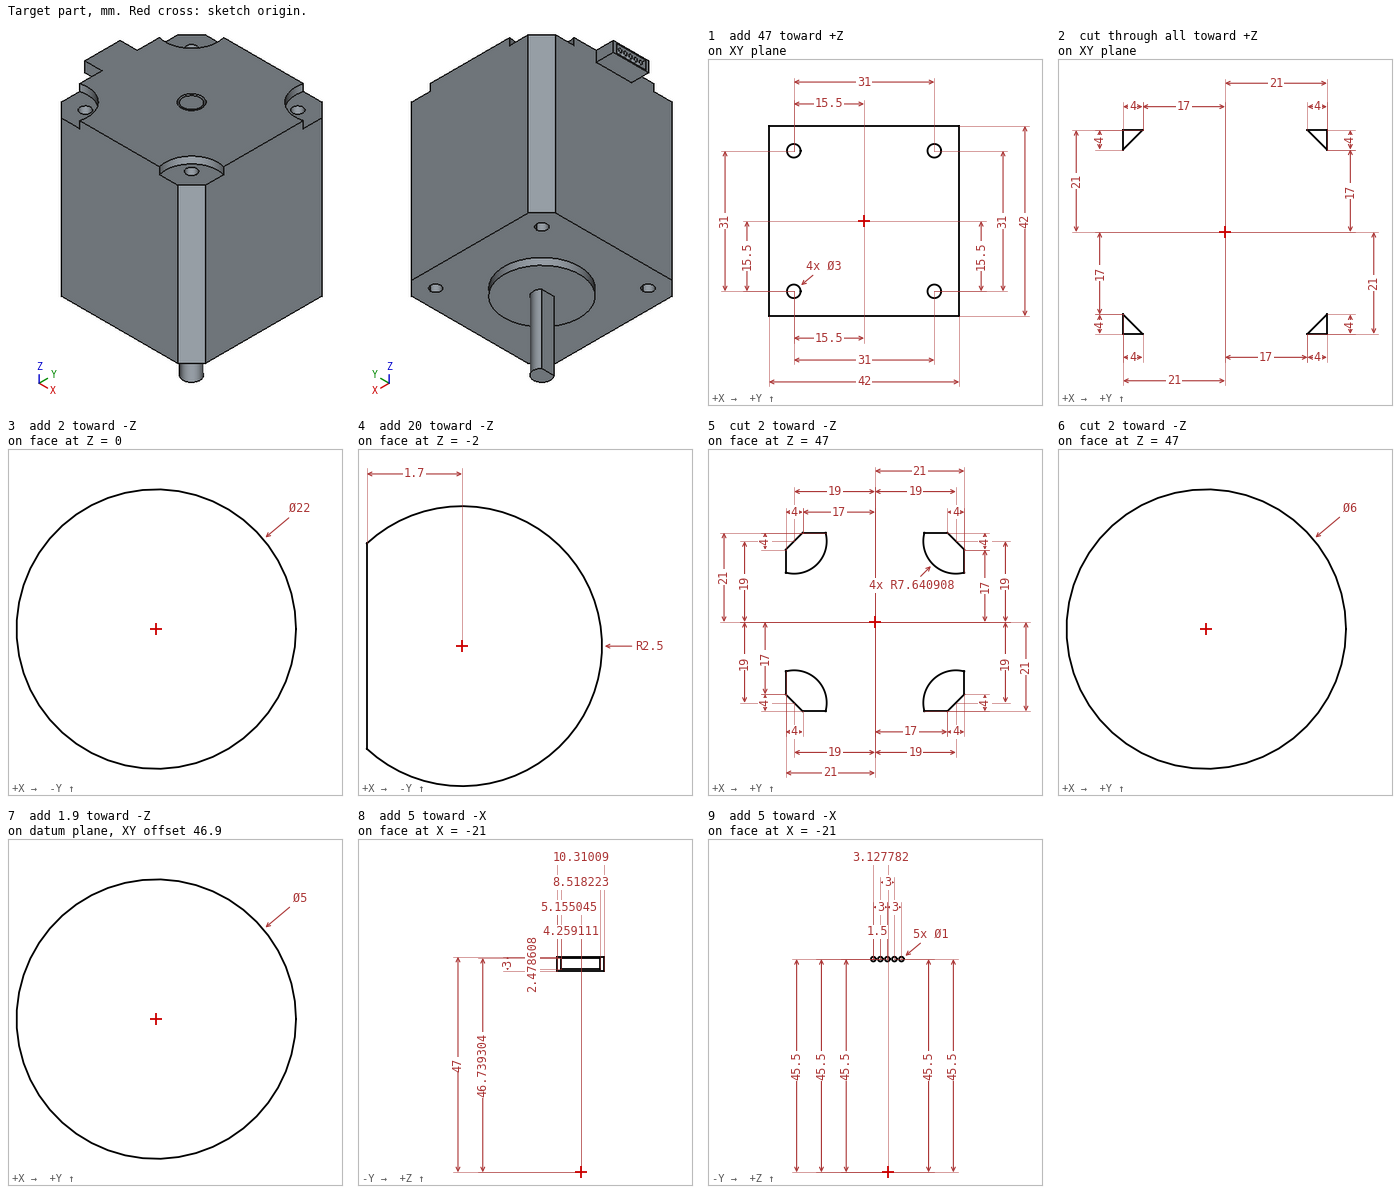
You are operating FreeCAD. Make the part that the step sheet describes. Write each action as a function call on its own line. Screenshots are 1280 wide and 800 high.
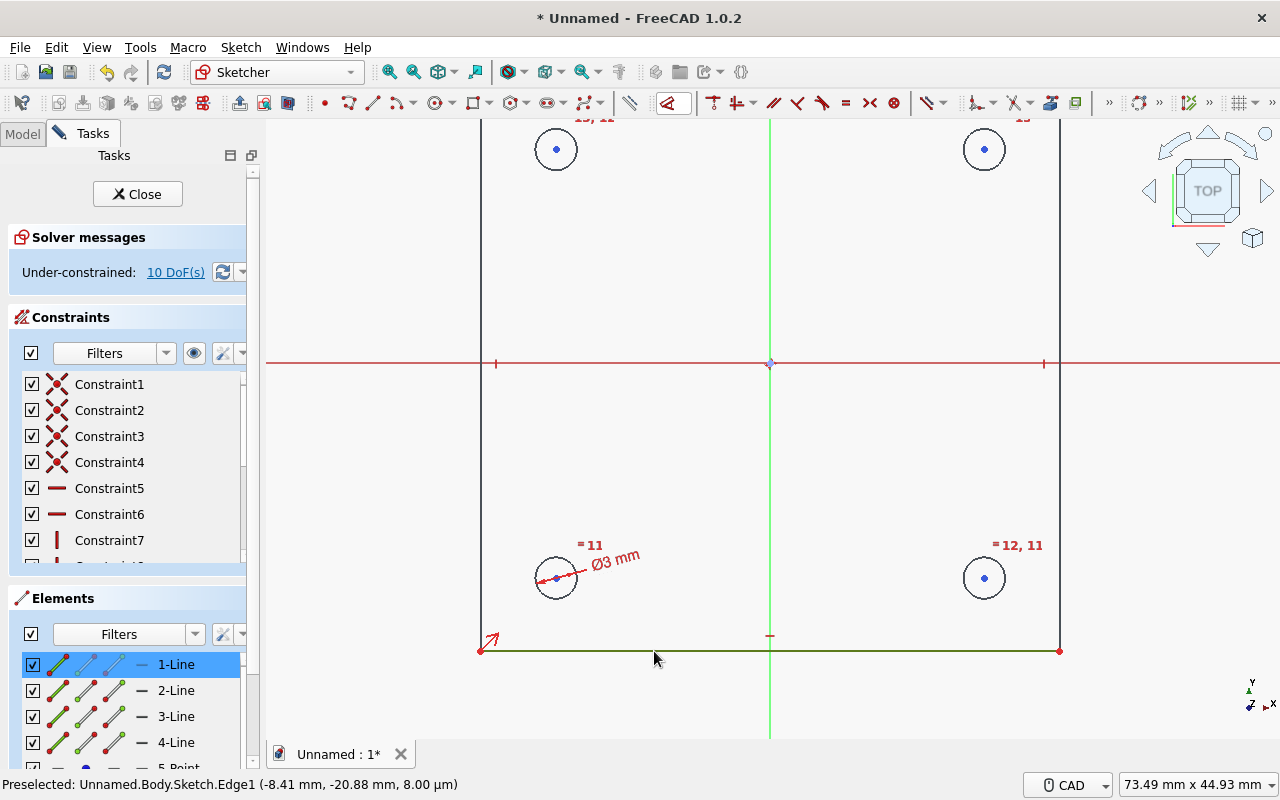
click(686, 104)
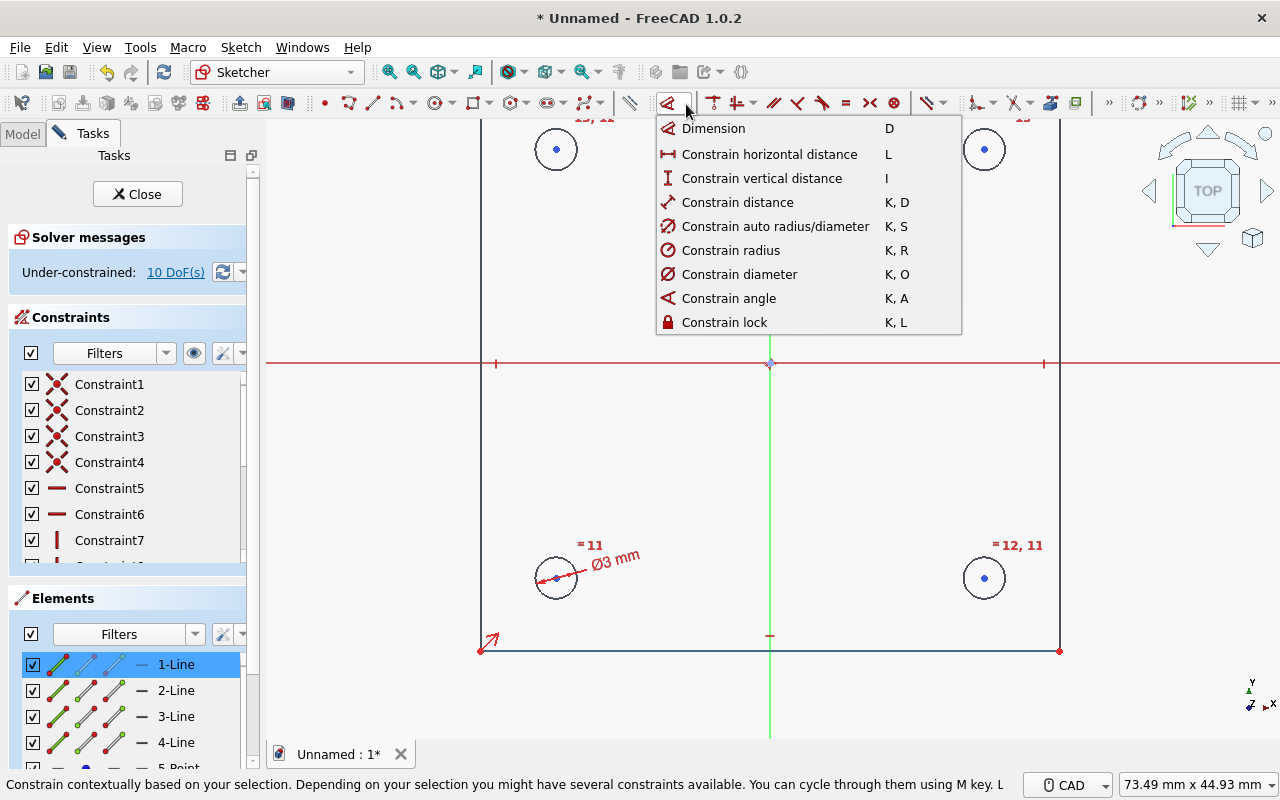
click(809, 154)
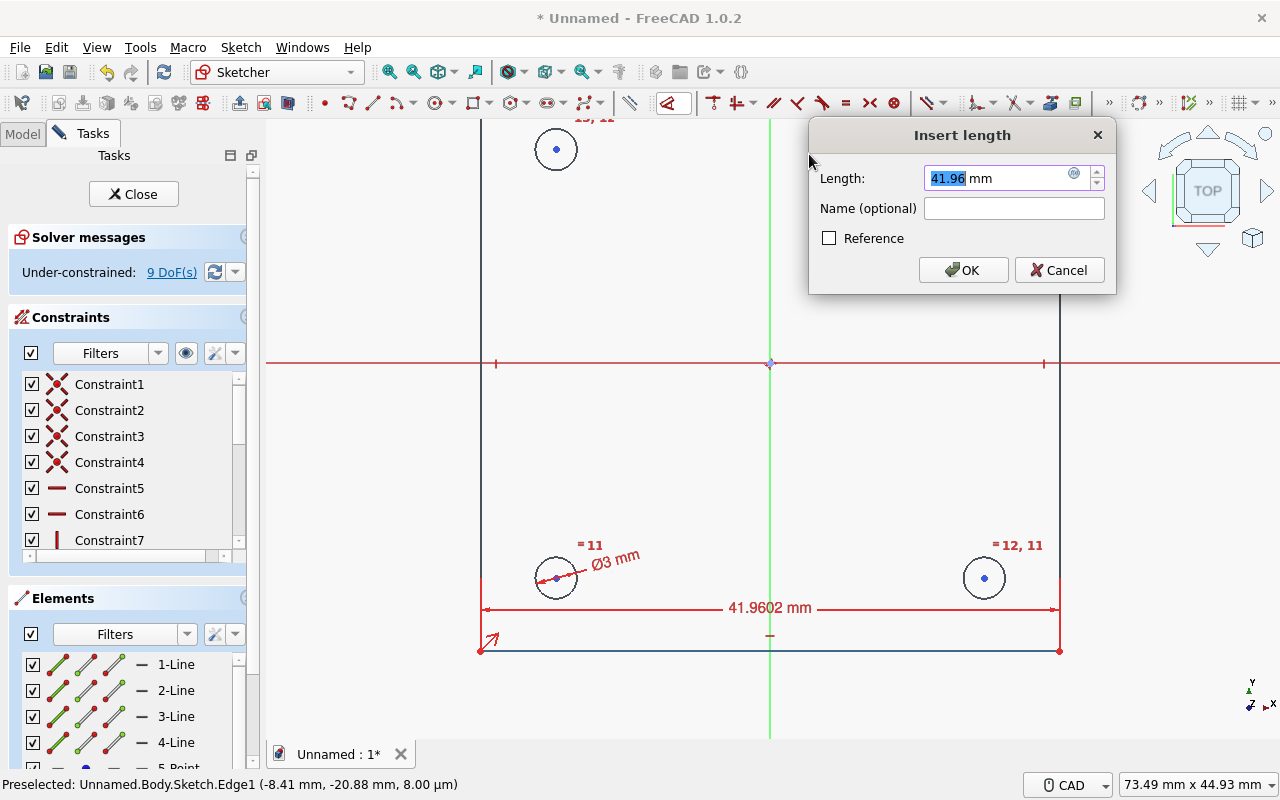
text(42)
key(Return)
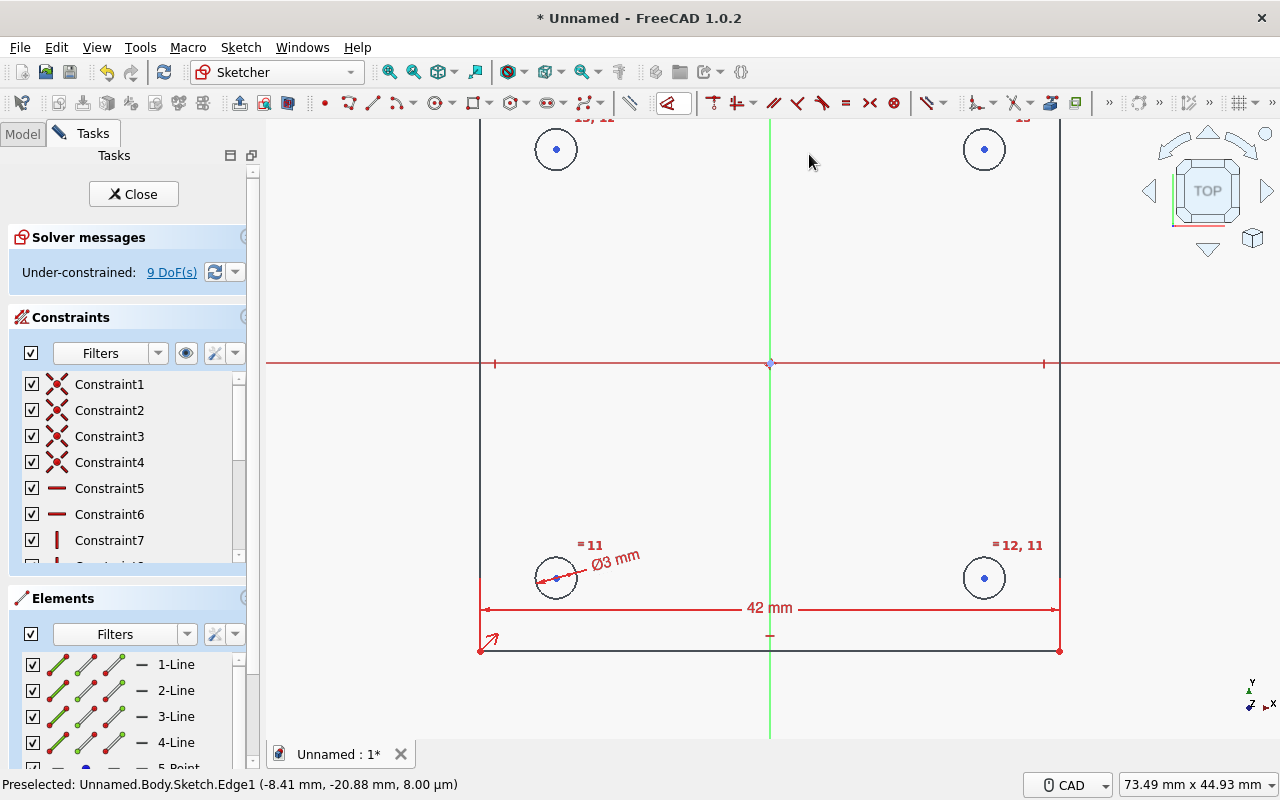
click(1060, 478)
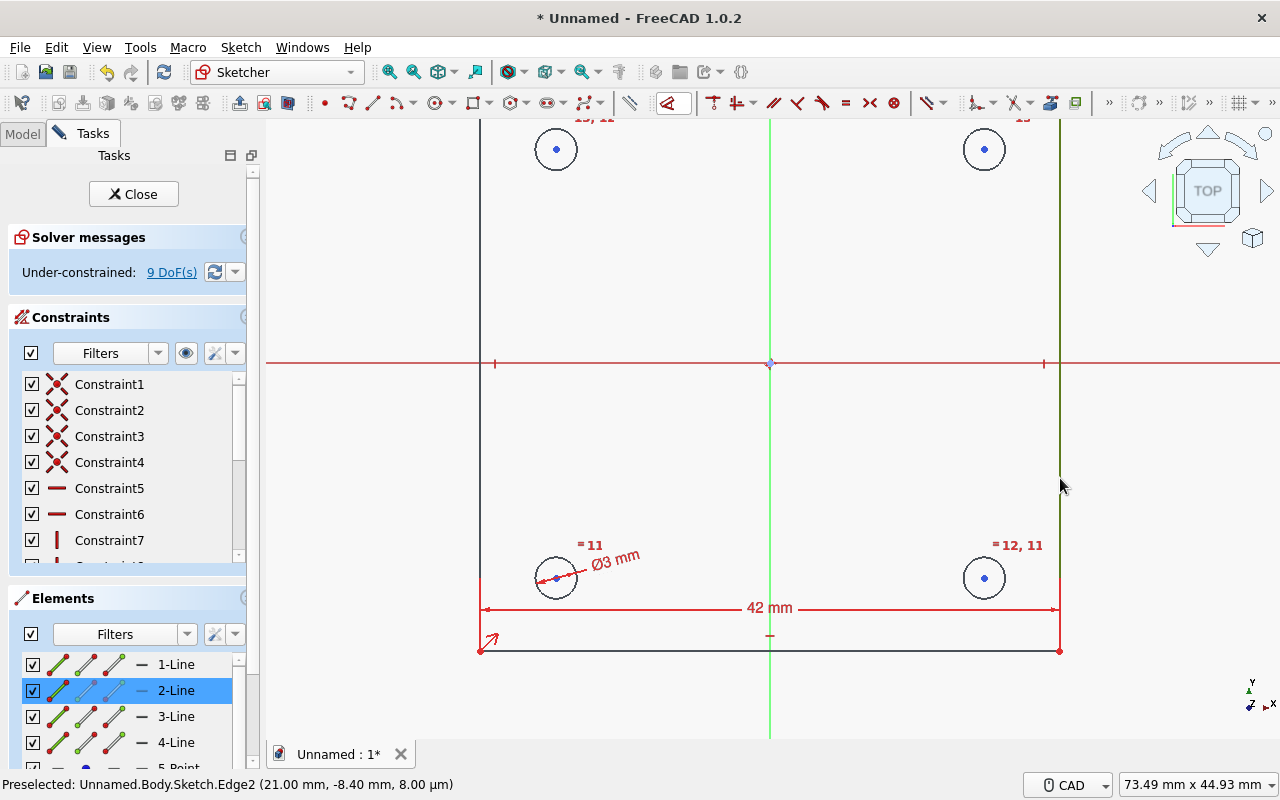
key(i)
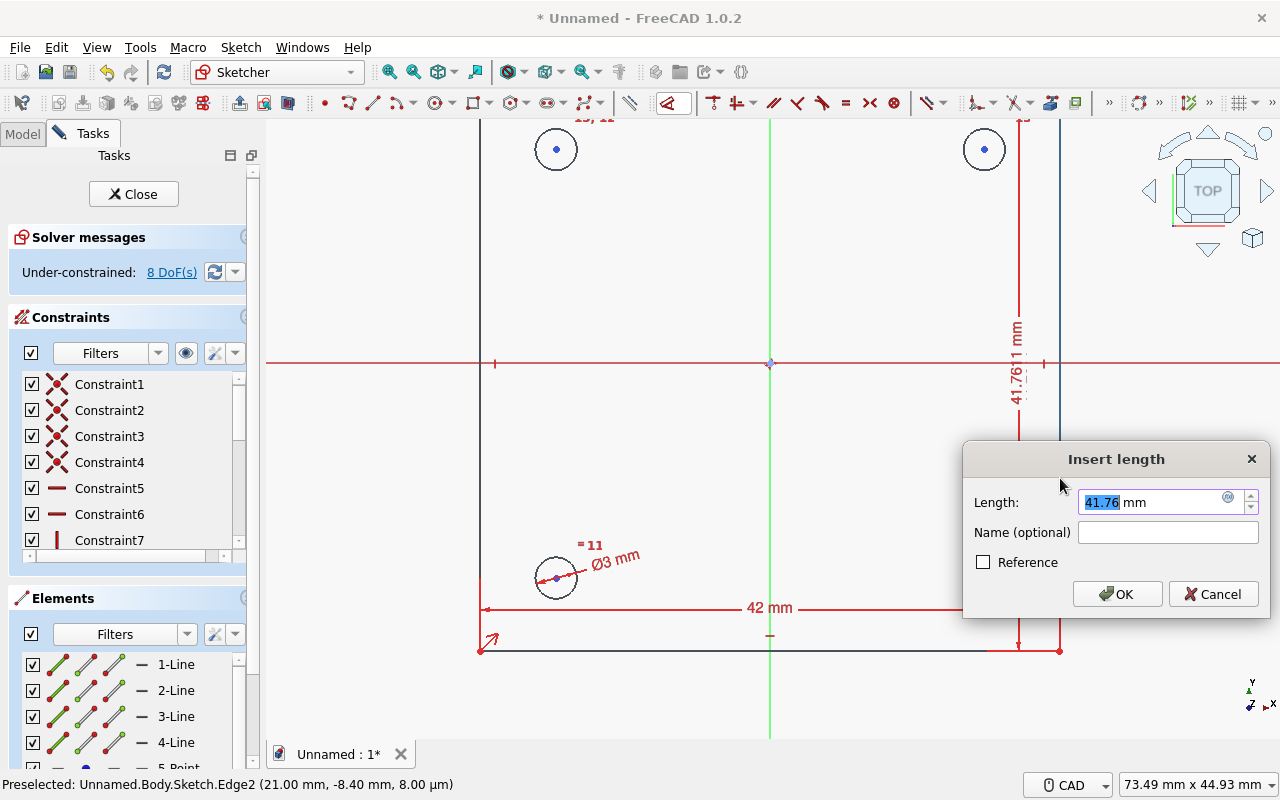
text(42)
key(Return)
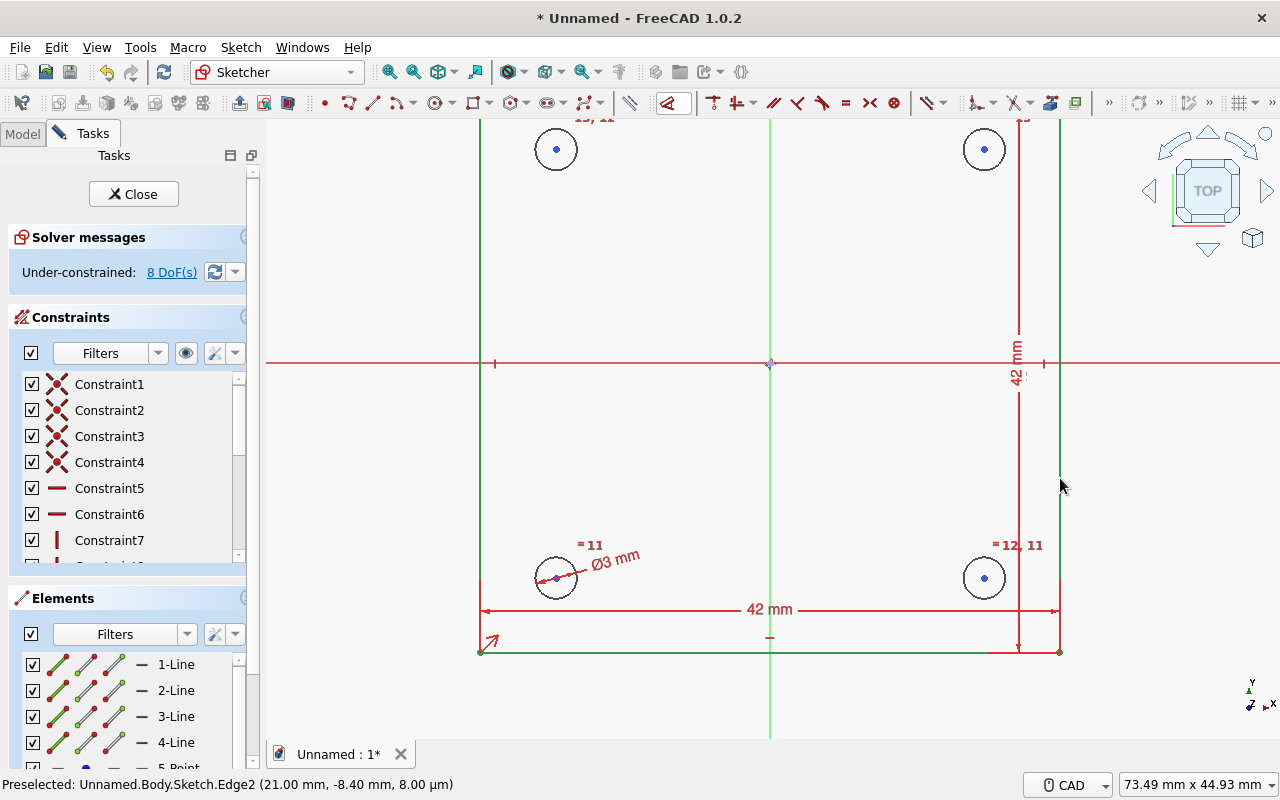
click(556, 578)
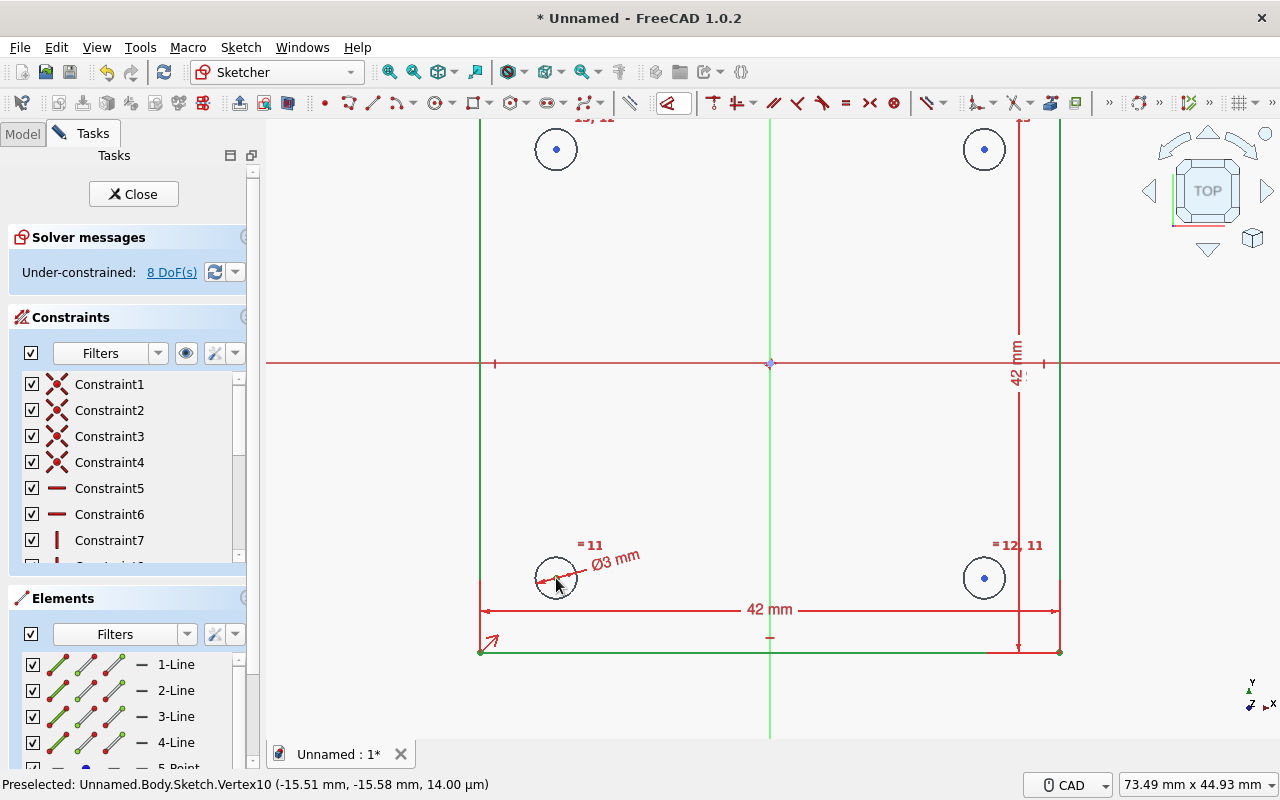
click(984, 578)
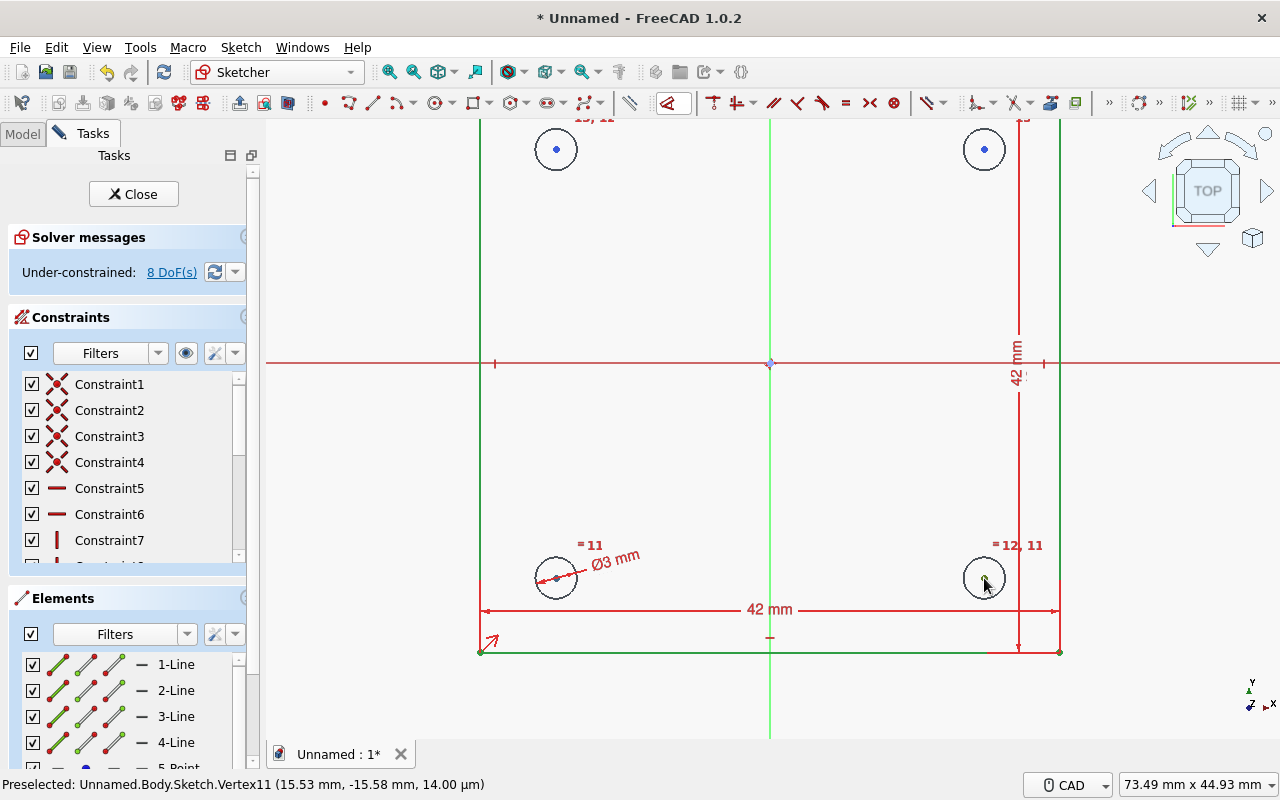
click(686, 104)